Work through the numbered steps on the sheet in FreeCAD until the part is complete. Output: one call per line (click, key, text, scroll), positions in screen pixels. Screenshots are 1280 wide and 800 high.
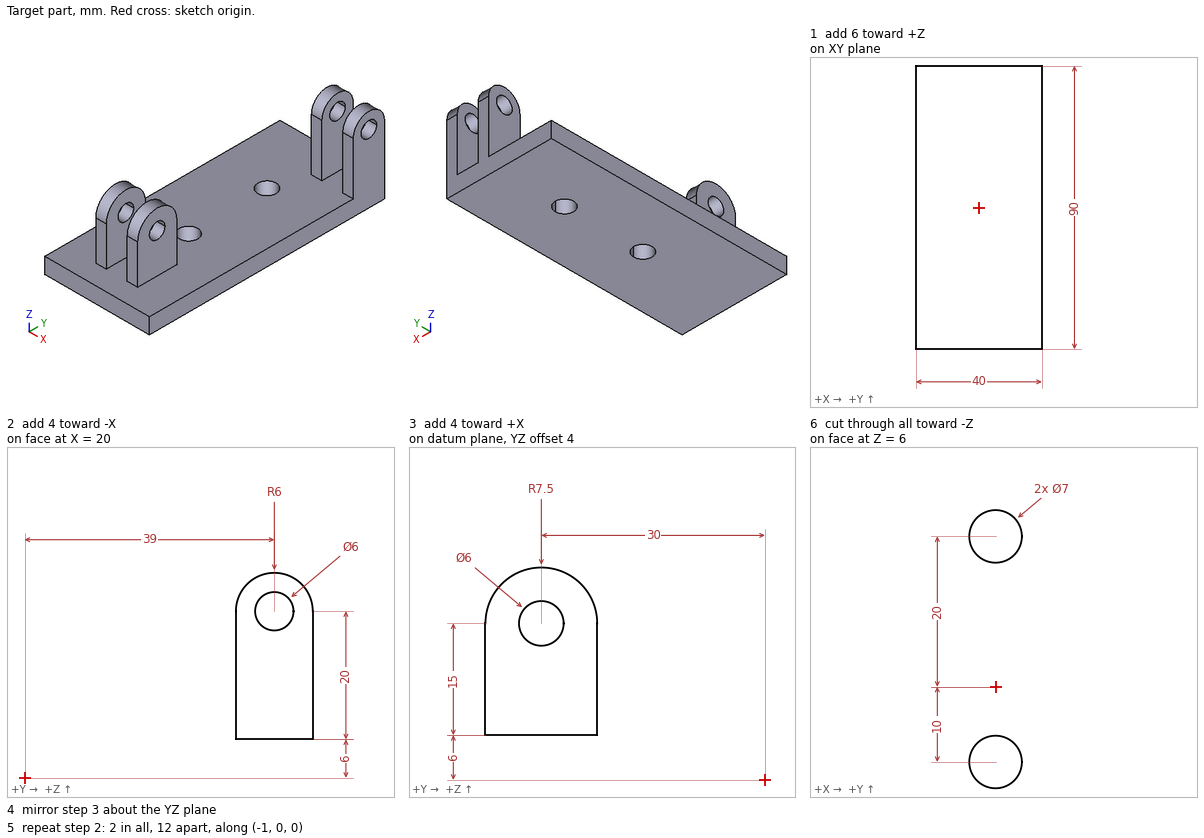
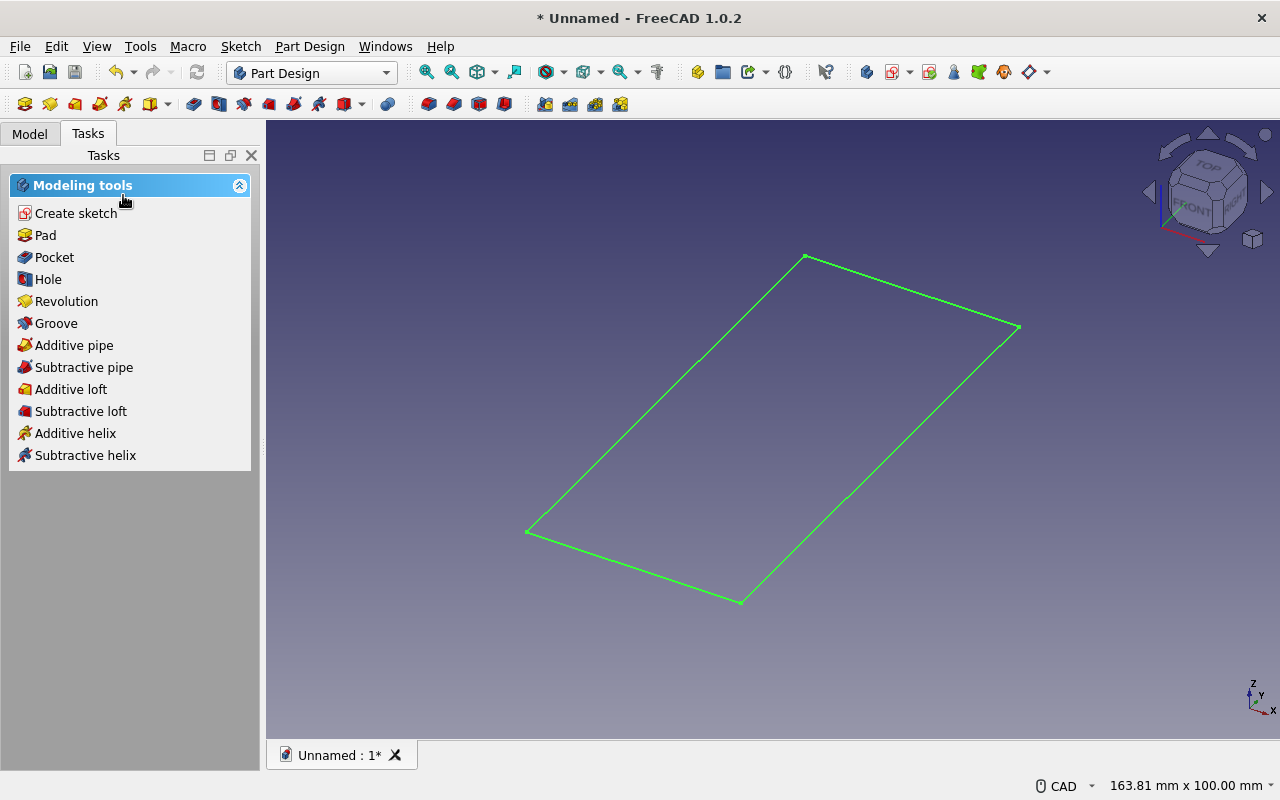
click(25, 104)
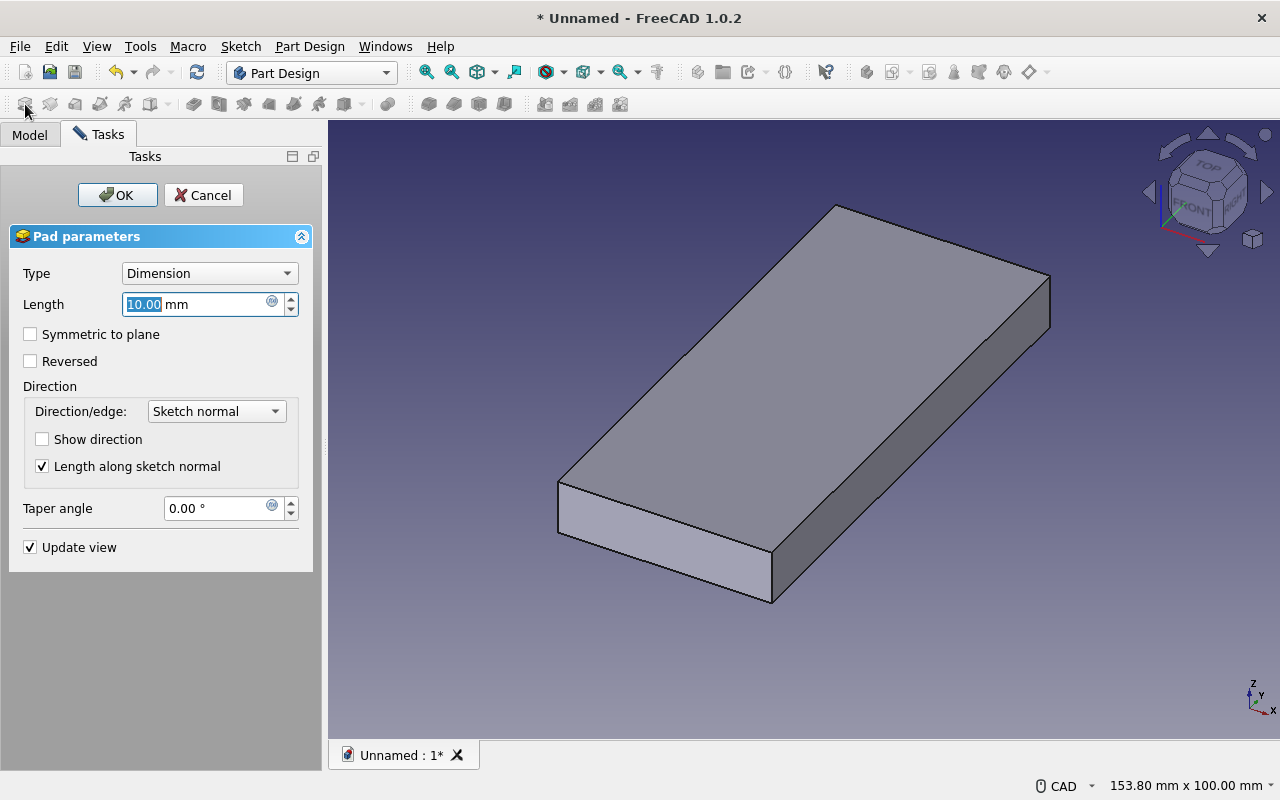
text(6)
key(Tab)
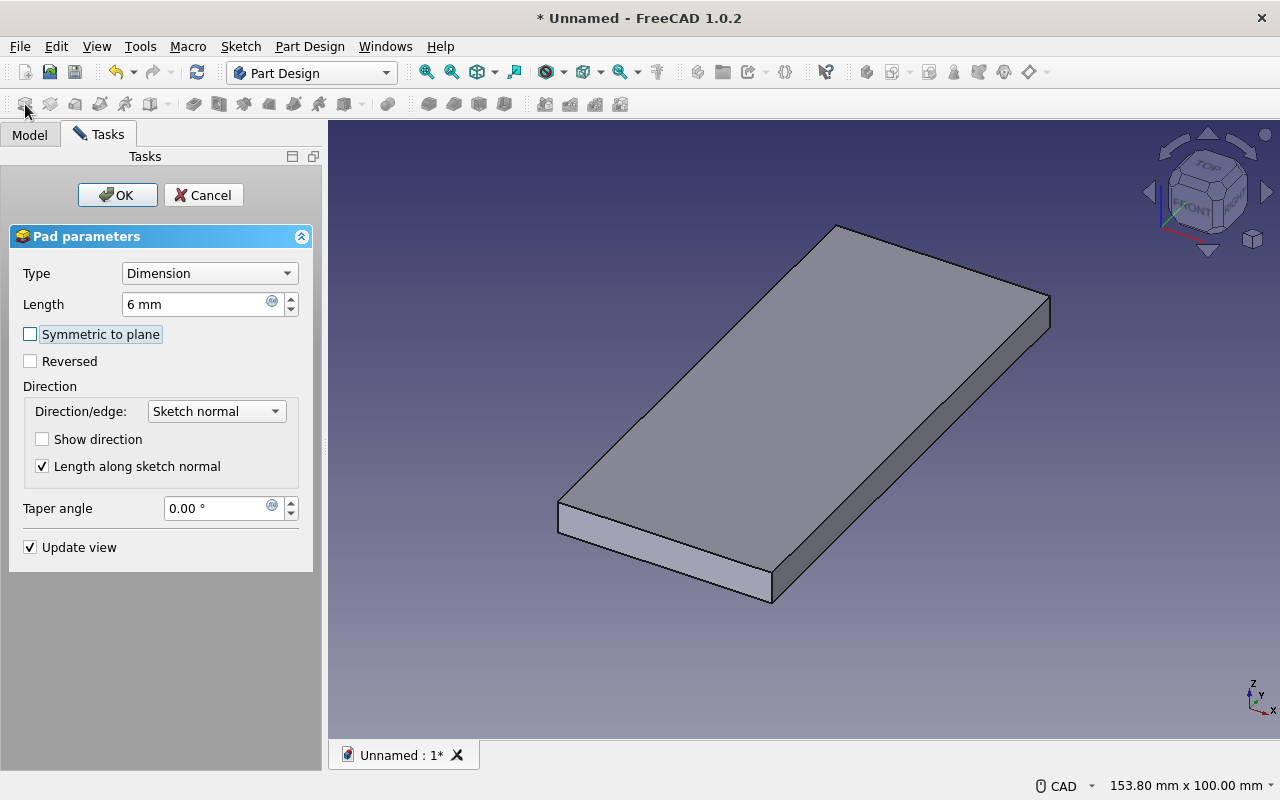
click(118, 195)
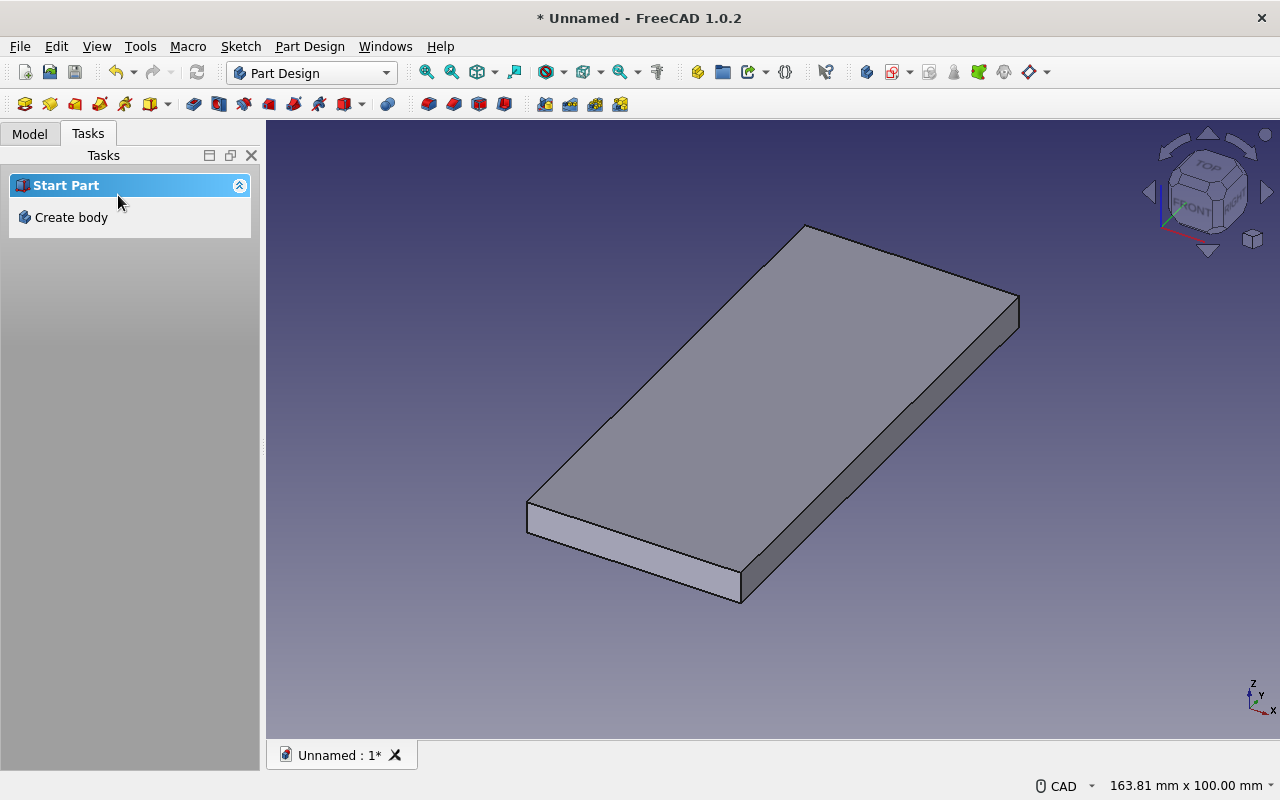
click(1000, 330)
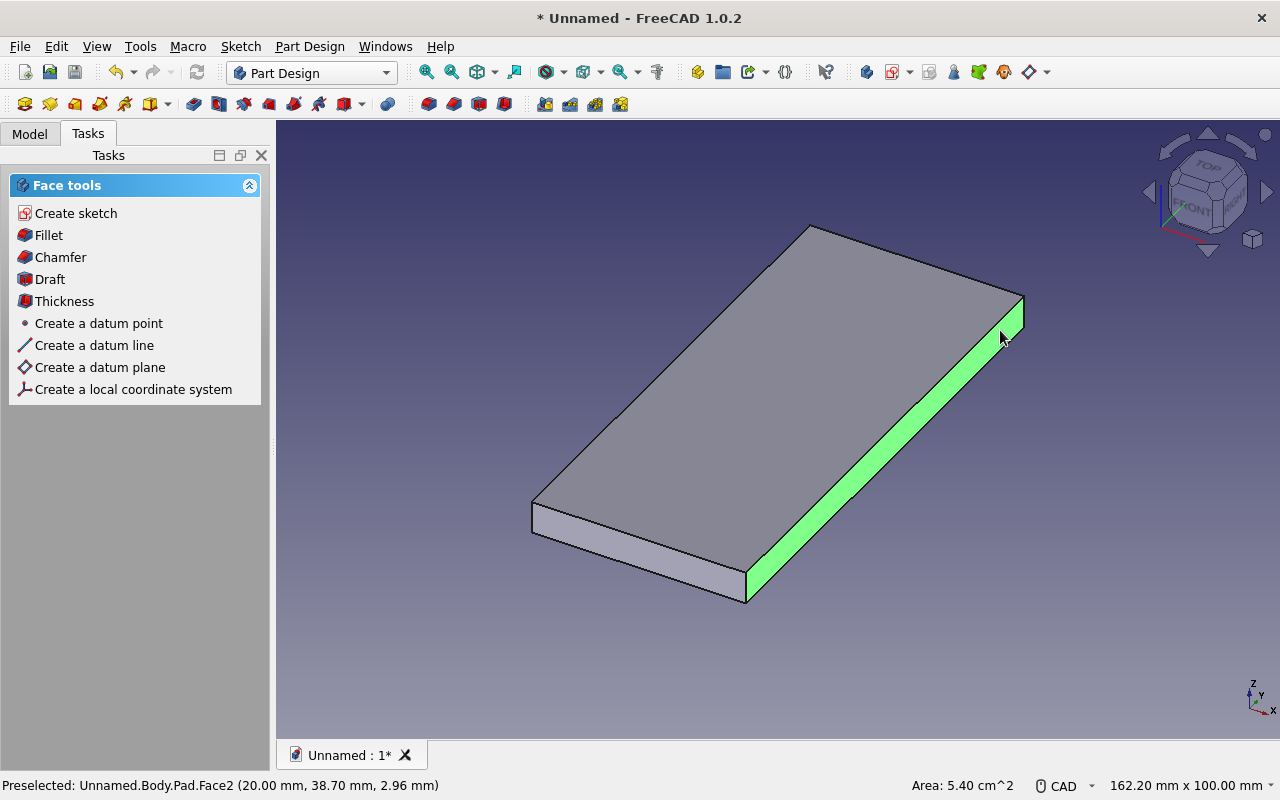
click(892, 72)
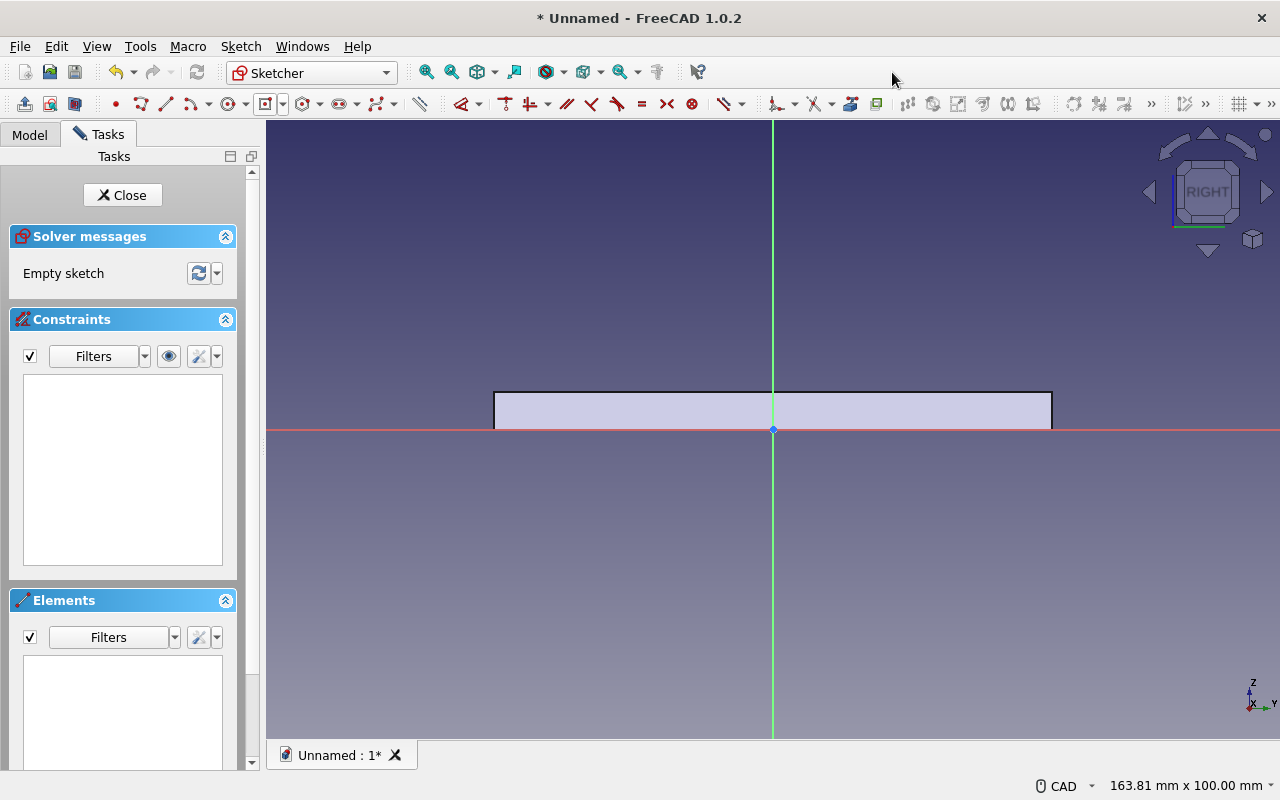
scroll(1115, 210, up, 3)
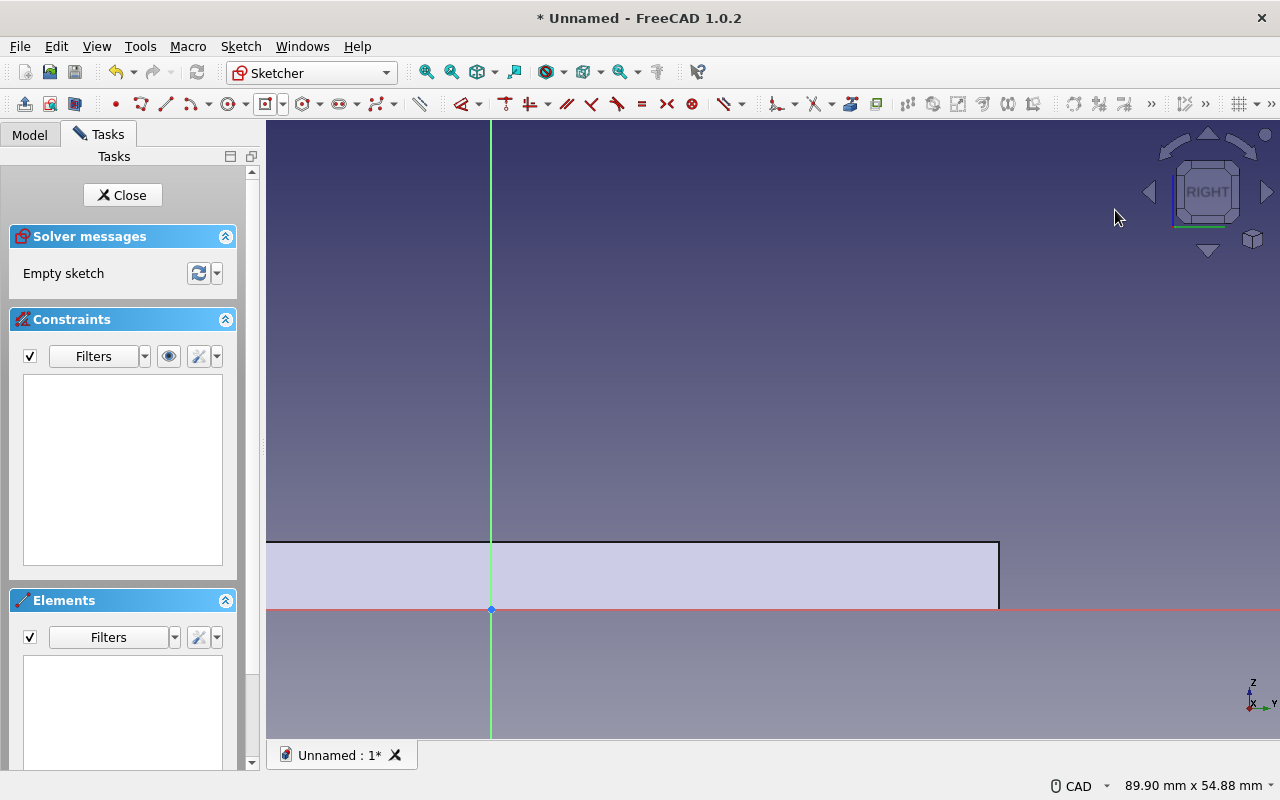
click(141, 104)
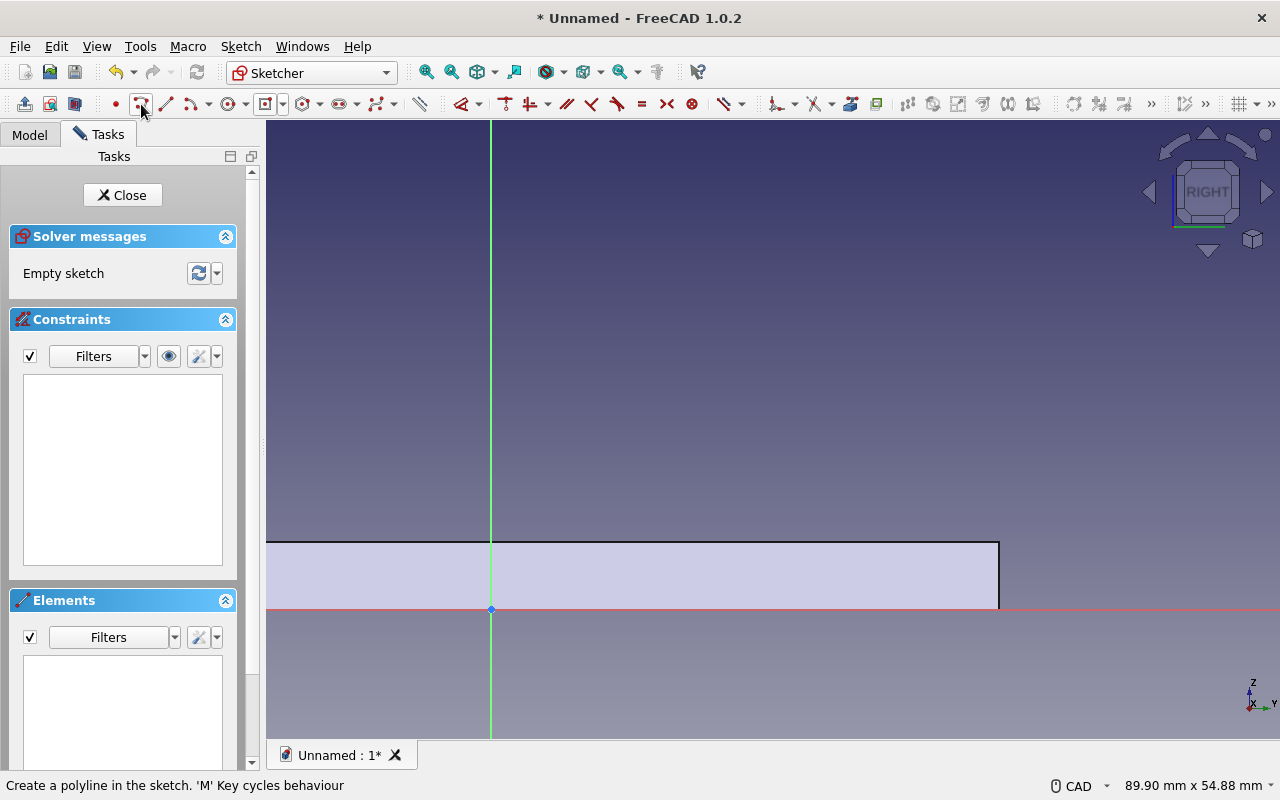
click(999, 317)
click(999, 542)
click(863, 542)
click(863, 317)
right_click(863, 317)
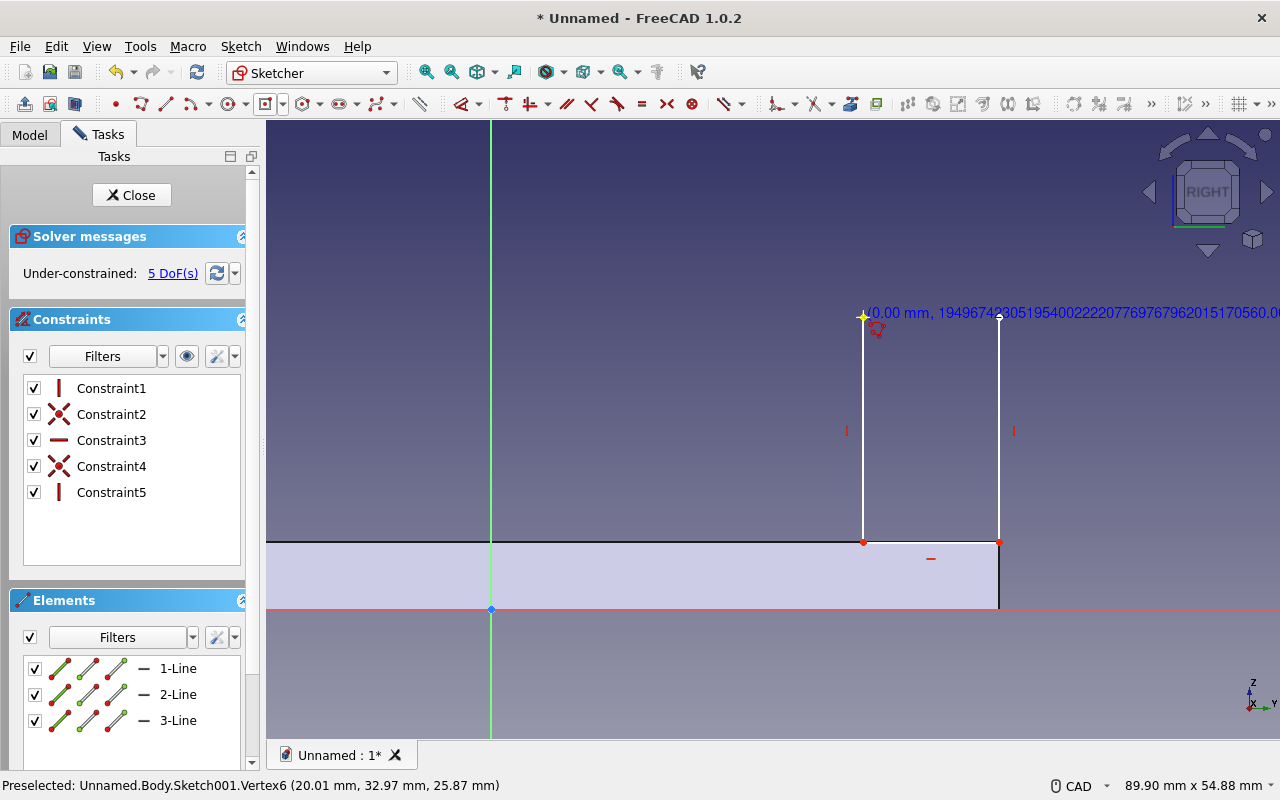
click(208, 104)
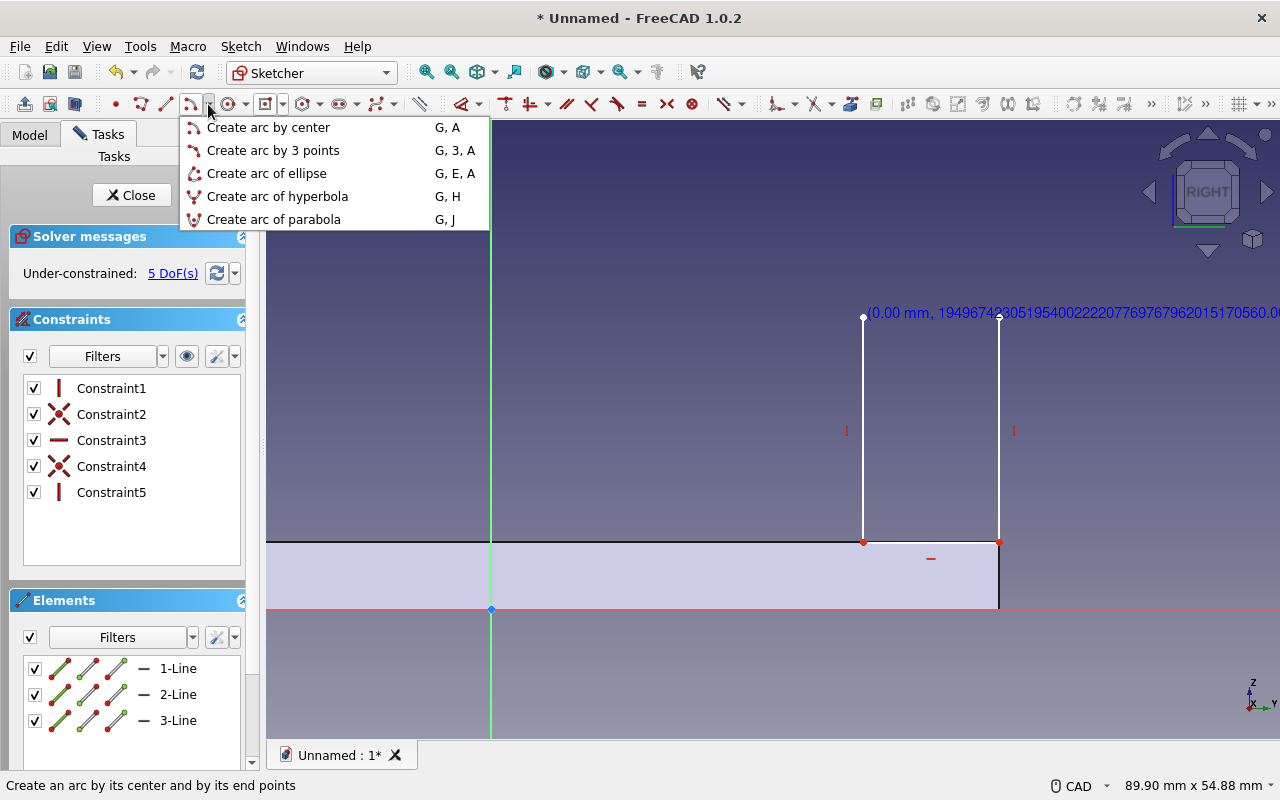
click(334, 150)